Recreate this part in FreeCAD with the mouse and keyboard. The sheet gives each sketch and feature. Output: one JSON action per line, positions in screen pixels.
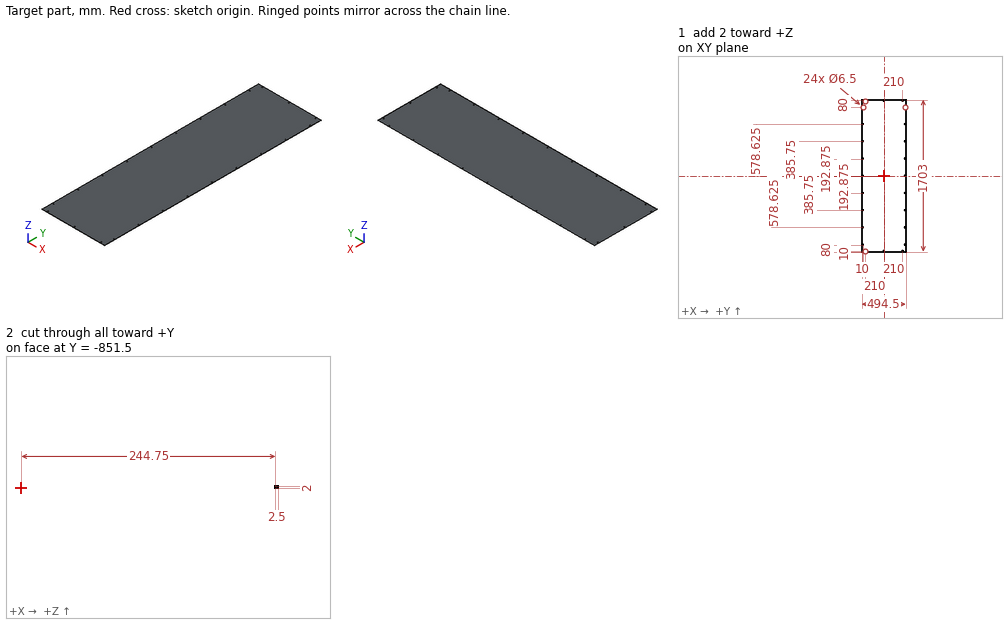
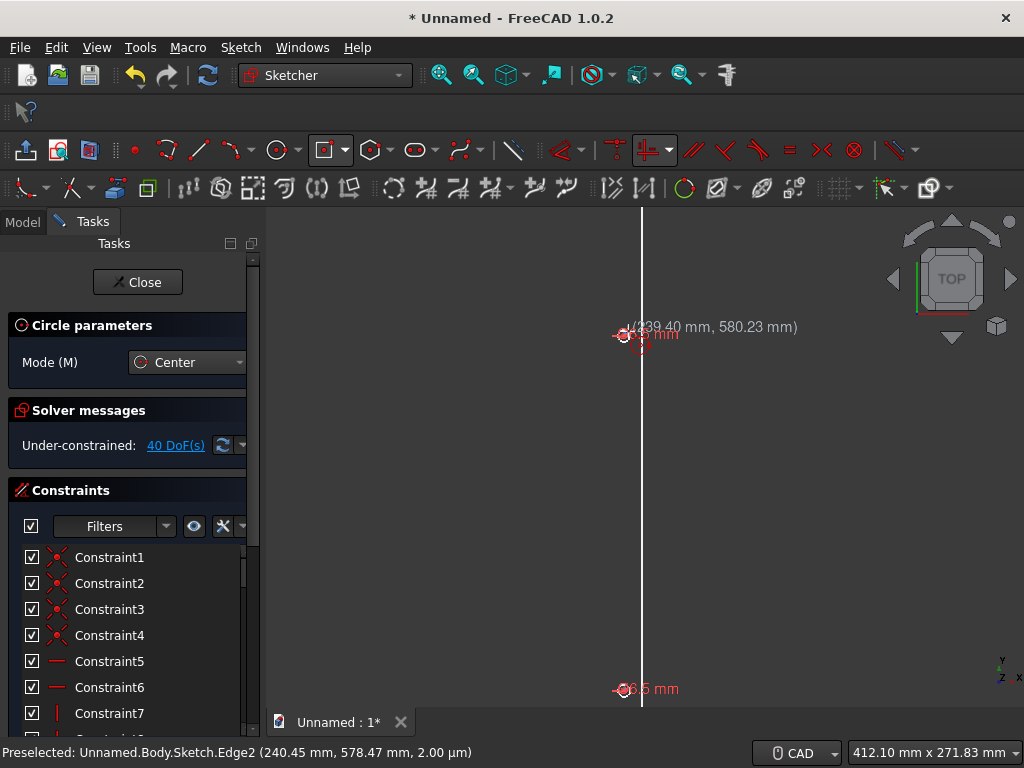
{"action": "scroll", "coordinate": [615, 363], "scroll_direction": "down", "scroll_amount": 12}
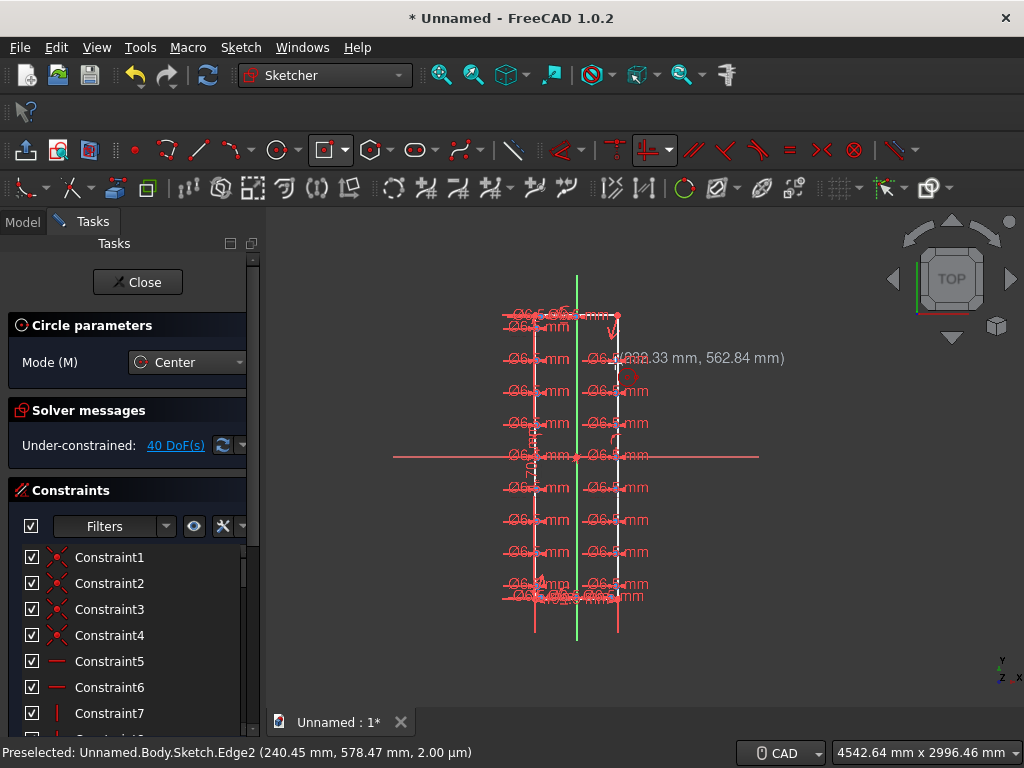
{"action": "scroll", "coordinate": [612, 317], "scroll_direction": "up", "scroll_amount": 19}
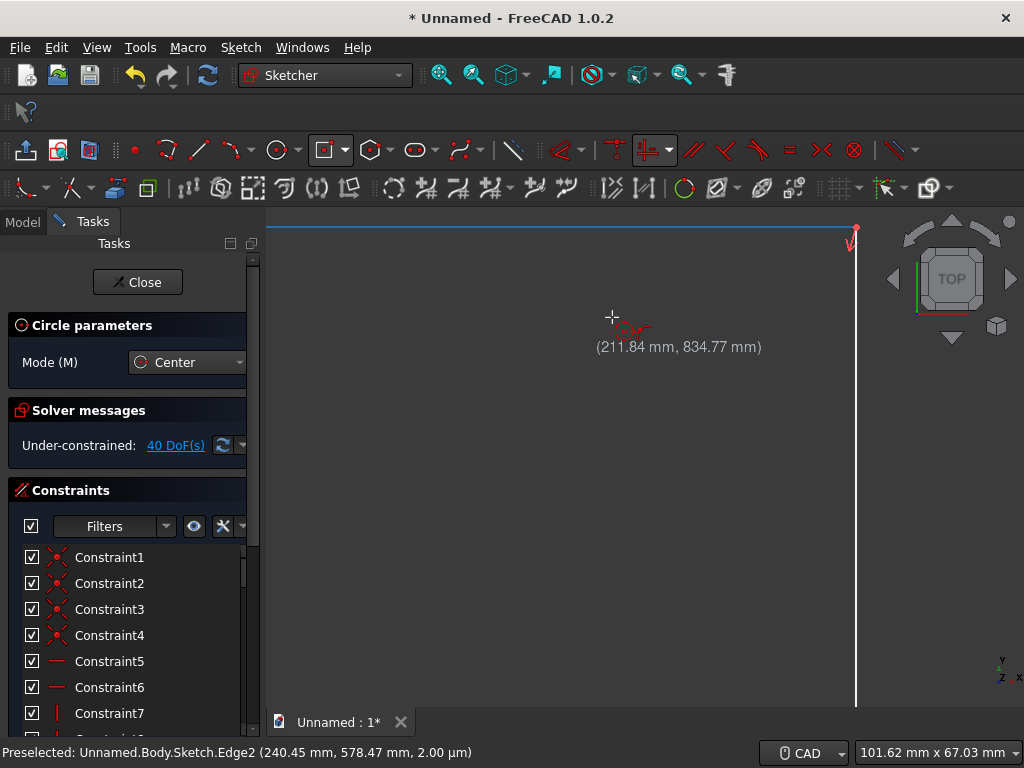
{"action": "scroll", "coordinate": [620, 285], "scroll_direction": "down", "scroll_amount": 18}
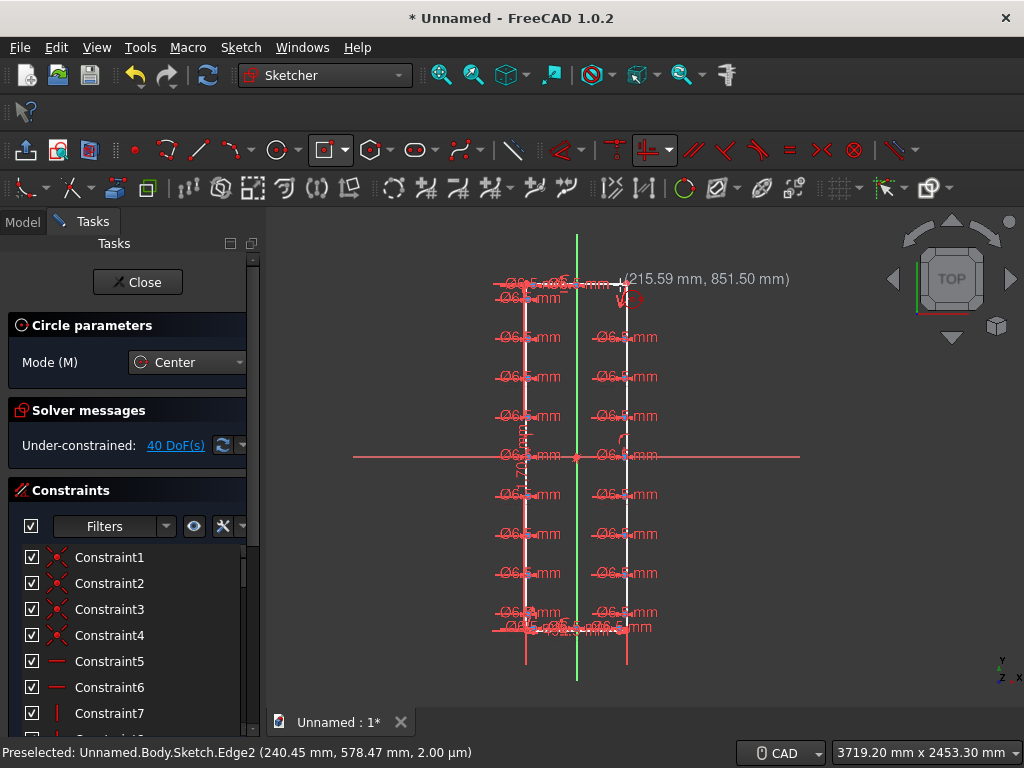
{"action": "scroll", "coordinate": [619, 286], "scroll_direction": "up", "scroll_amount": 11}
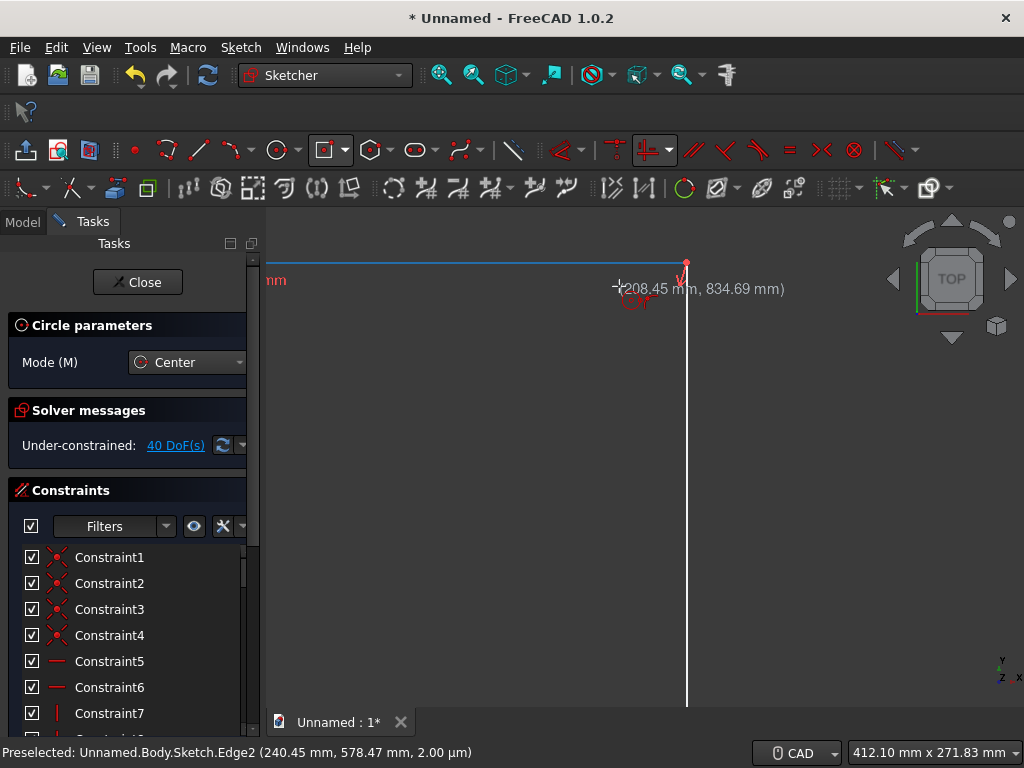
{"action": "left_click", "coordinate": [618, 281]}
{"action": "mouse_move", "coordinate": [622, 277]}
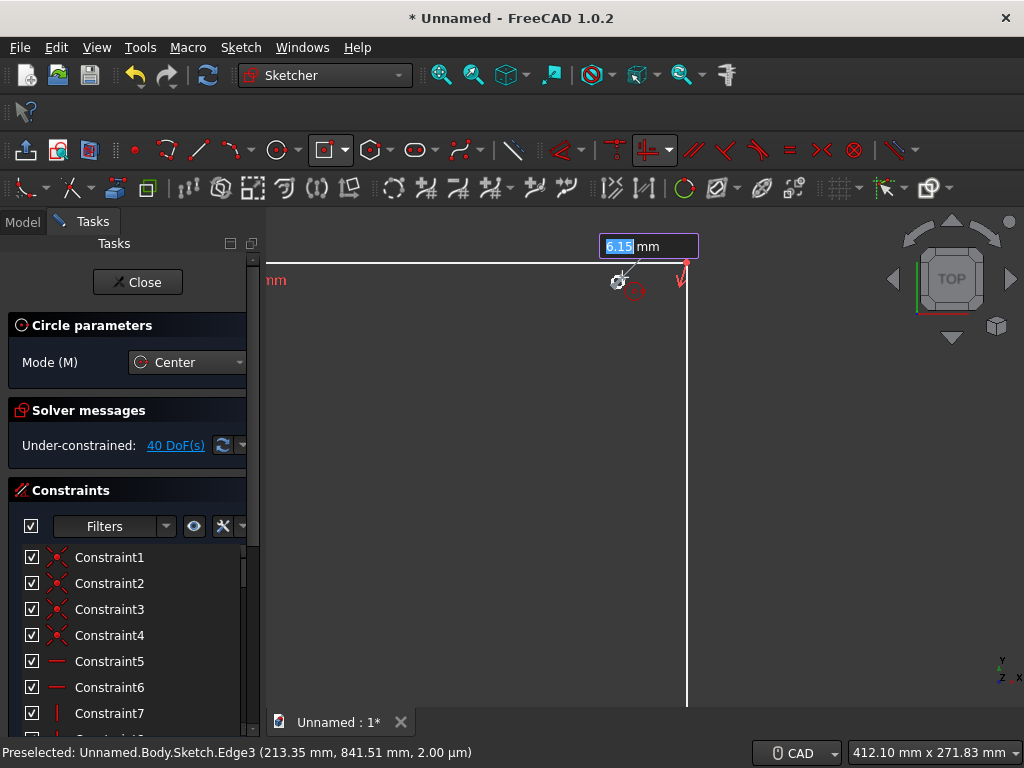
{"action": "type", "text": "6.5"}
{"action": "key", "text": "Return"}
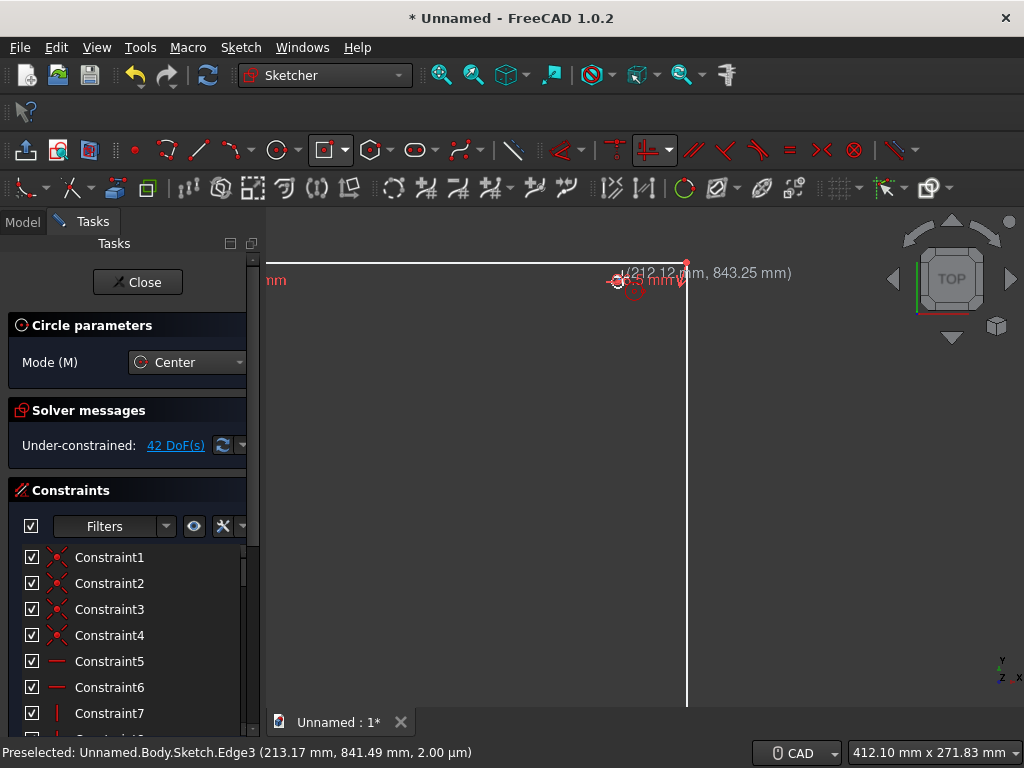
{"action": "scroll", "coordinate": [668, 410], "scroll_direction": "up", "scroll_amount": 7}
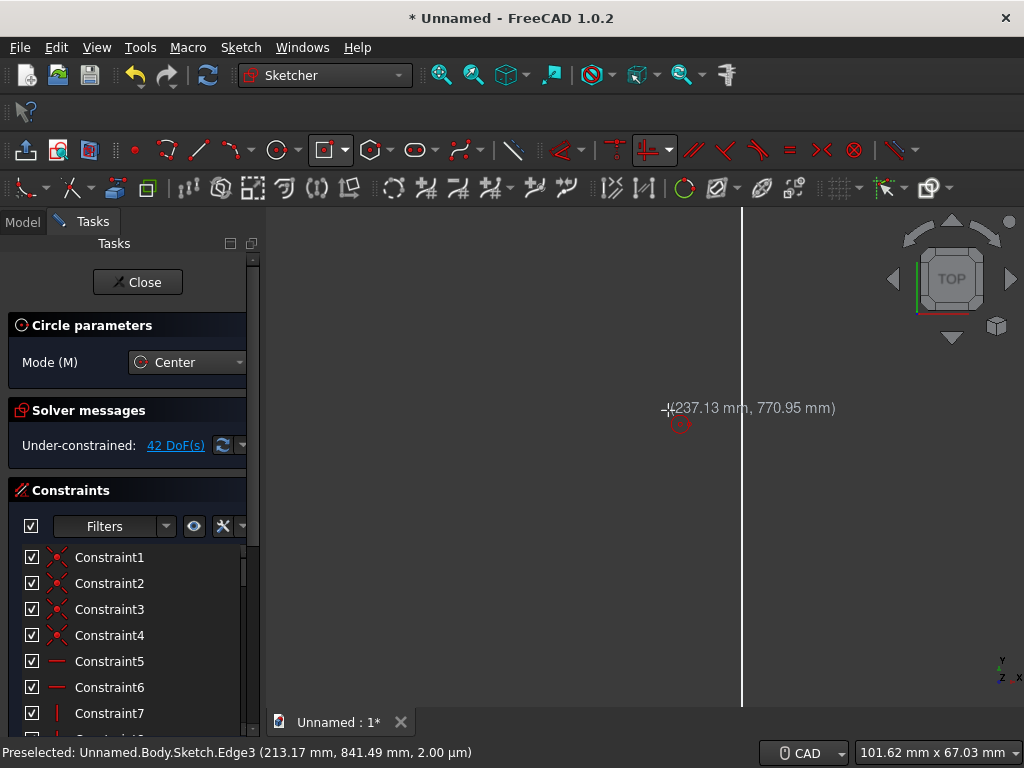
{"action": "scroll", "coordinate": [624, 297], "scroll_direction": "down", "scroll_amount": 18}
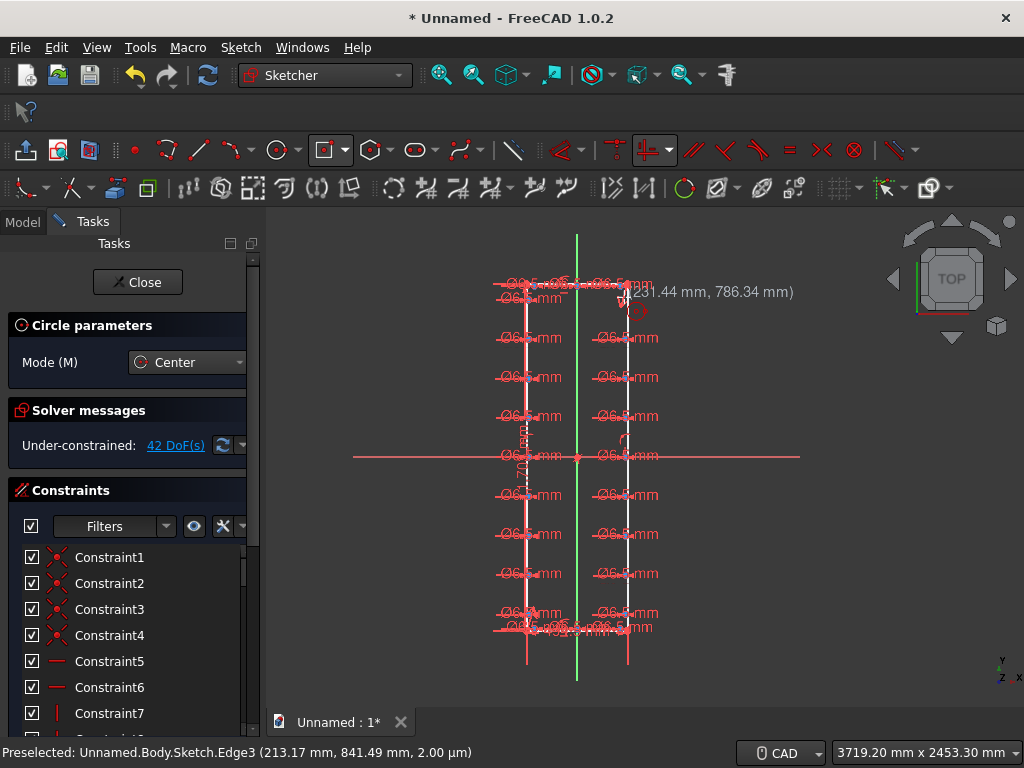
{"action": "scroll", "coordinate": [626, 300], "scroll_direction": "up", "scroll_amount": 11}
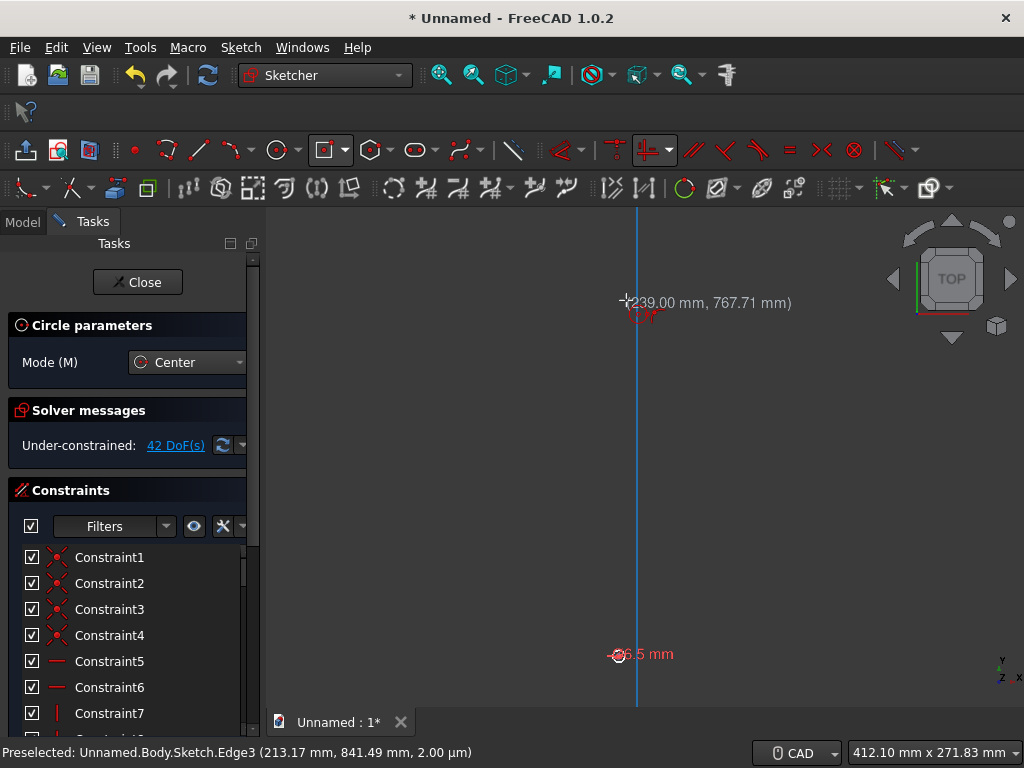
{"action": "left_click", "coordinate": [619, 301]}
{"action": "mouse_move", "coordinate": [623, 296]}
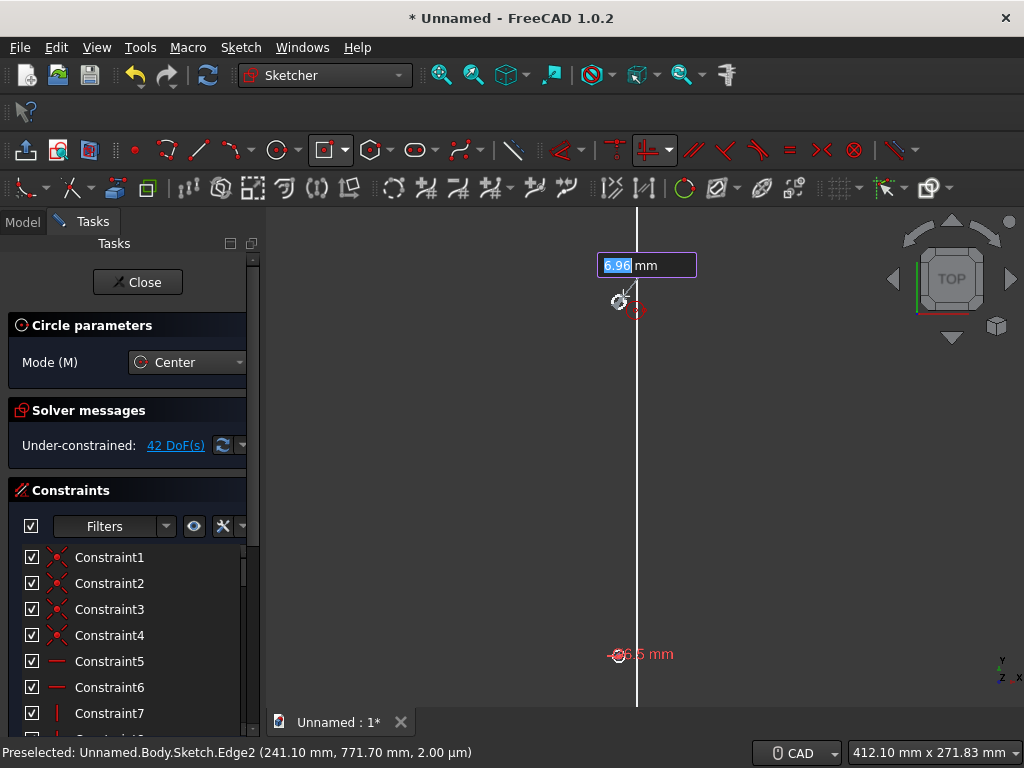
{"action": "type", "text": "6.5"}
{"action": "key", "text": "Return"}
{"action": "key", "text": "Escape"}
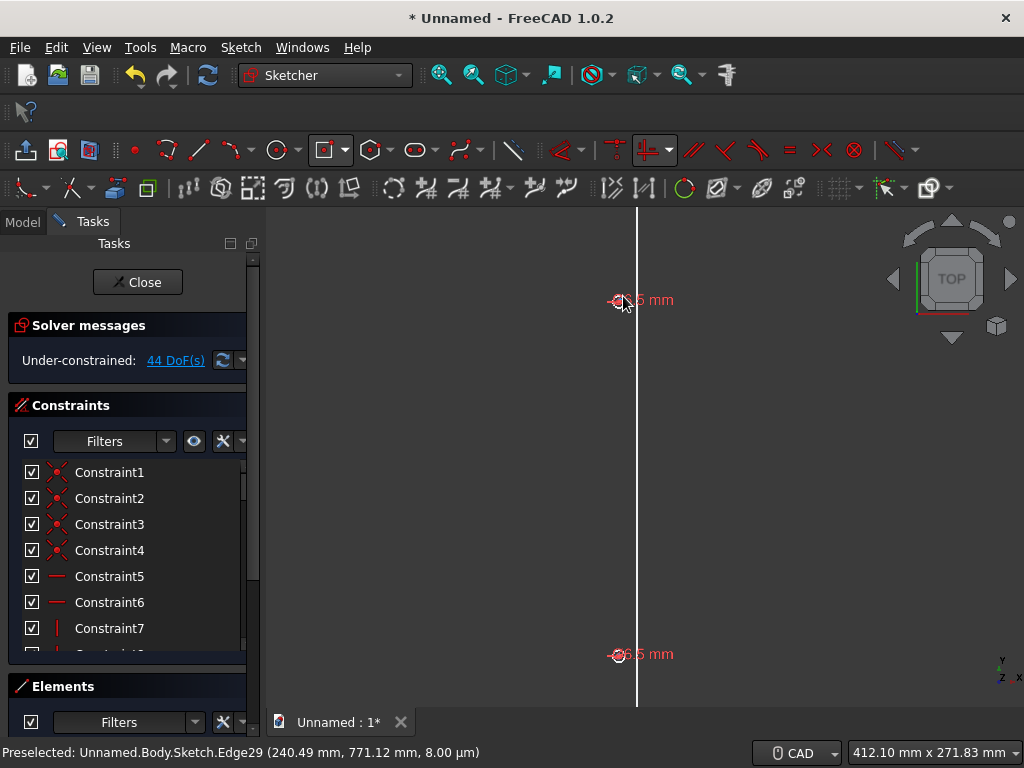
{"action": "scroll", "coordinate": [616, 331], "scroll_direction": "down", "scroll_amount": 12}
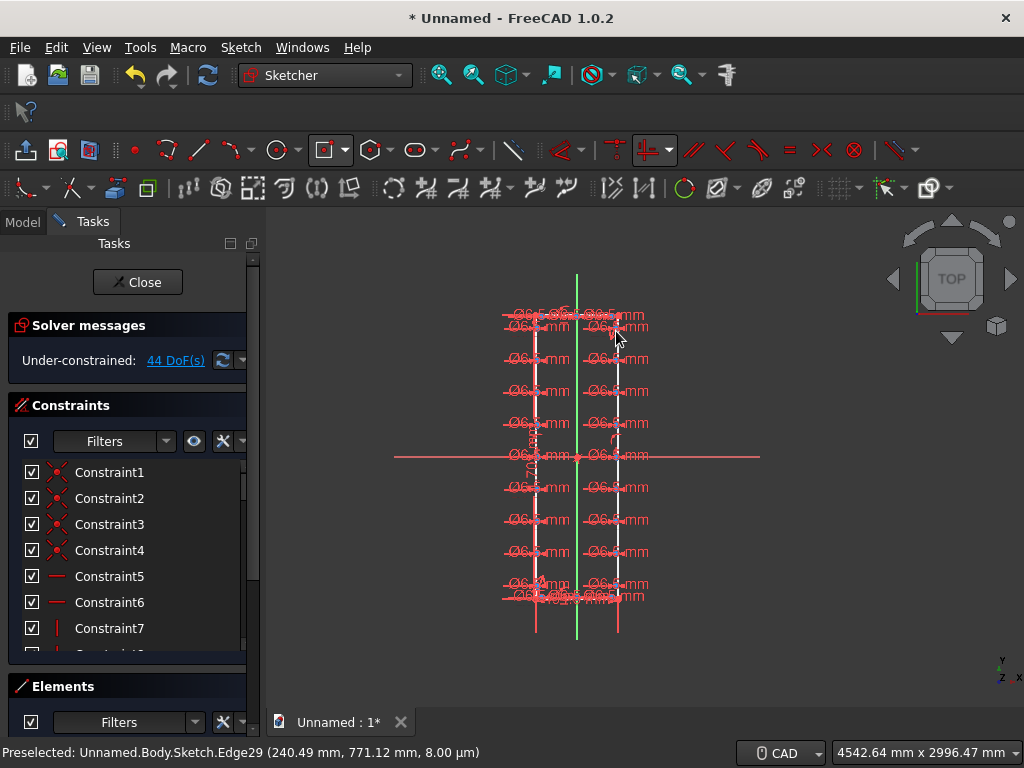
{"action": "left_click", "coordinate": [538, 586]}